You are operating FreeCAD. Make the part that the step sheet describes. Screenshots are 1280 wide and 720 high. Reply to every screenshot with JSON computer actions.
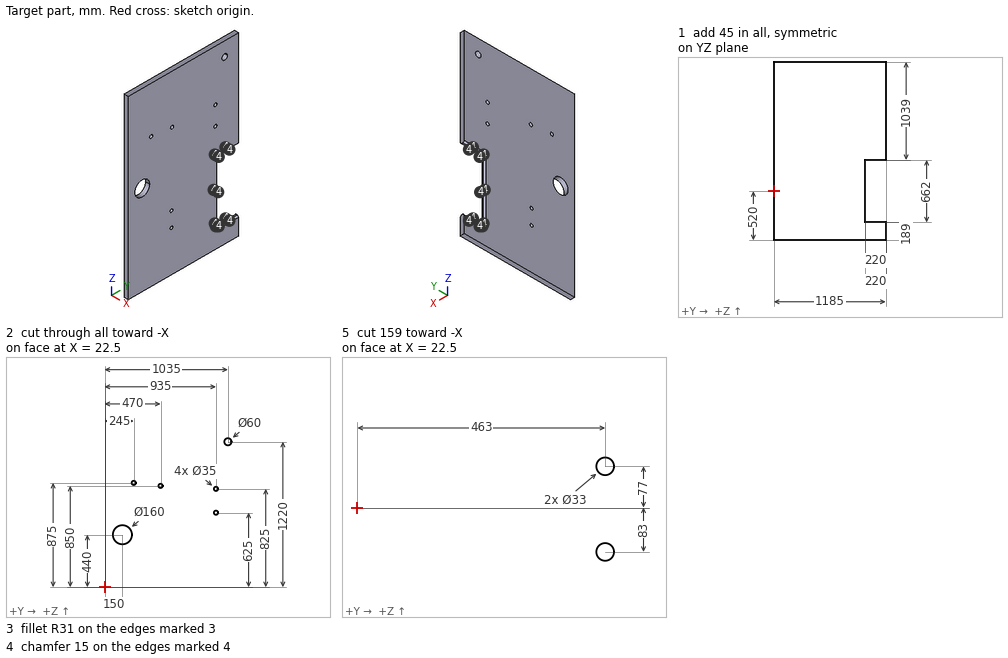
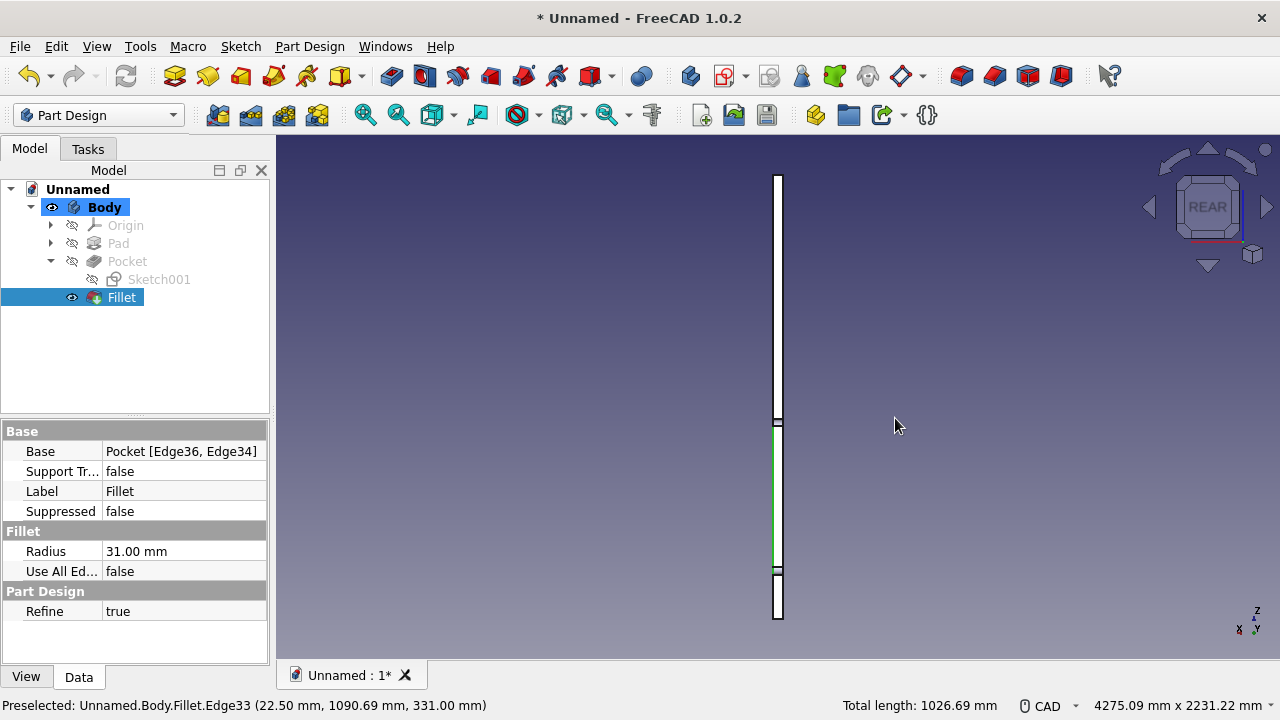
{"action": "left_click", "coordinate": [783, 496], "text": "ctrl"}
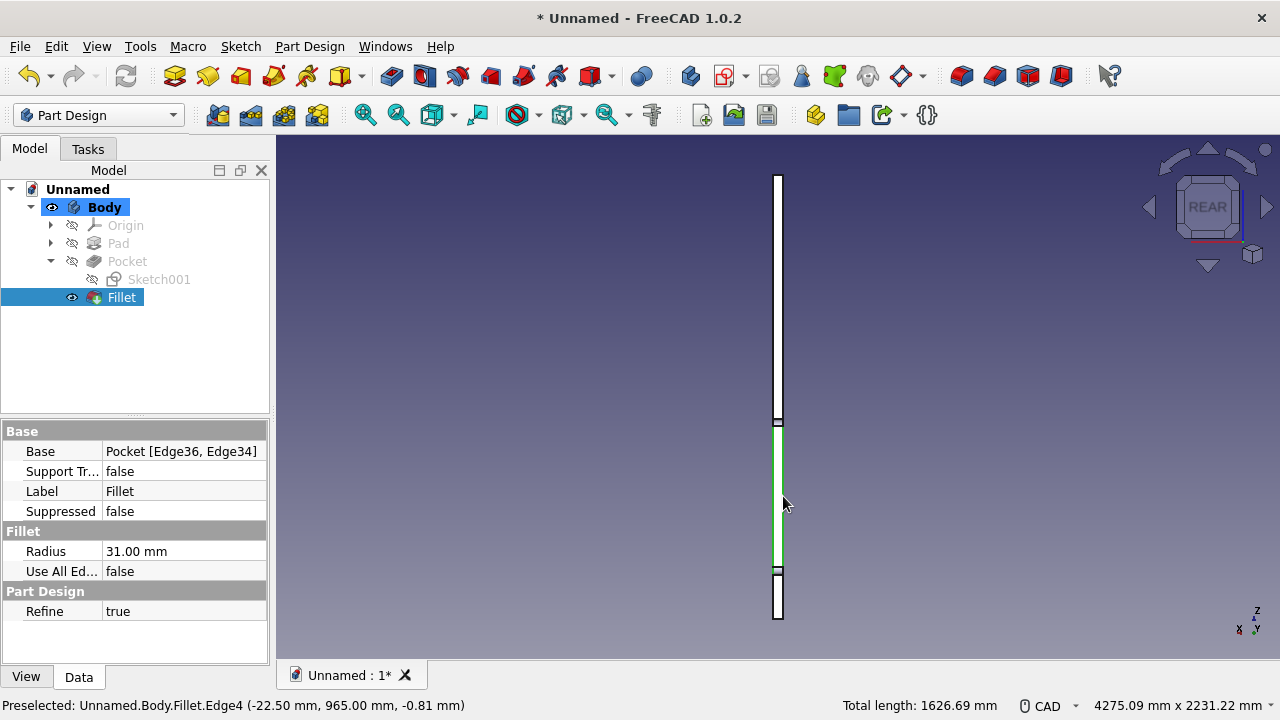
{"action": "left_click", "coordinate": [783, 425], "text": "ctrl"}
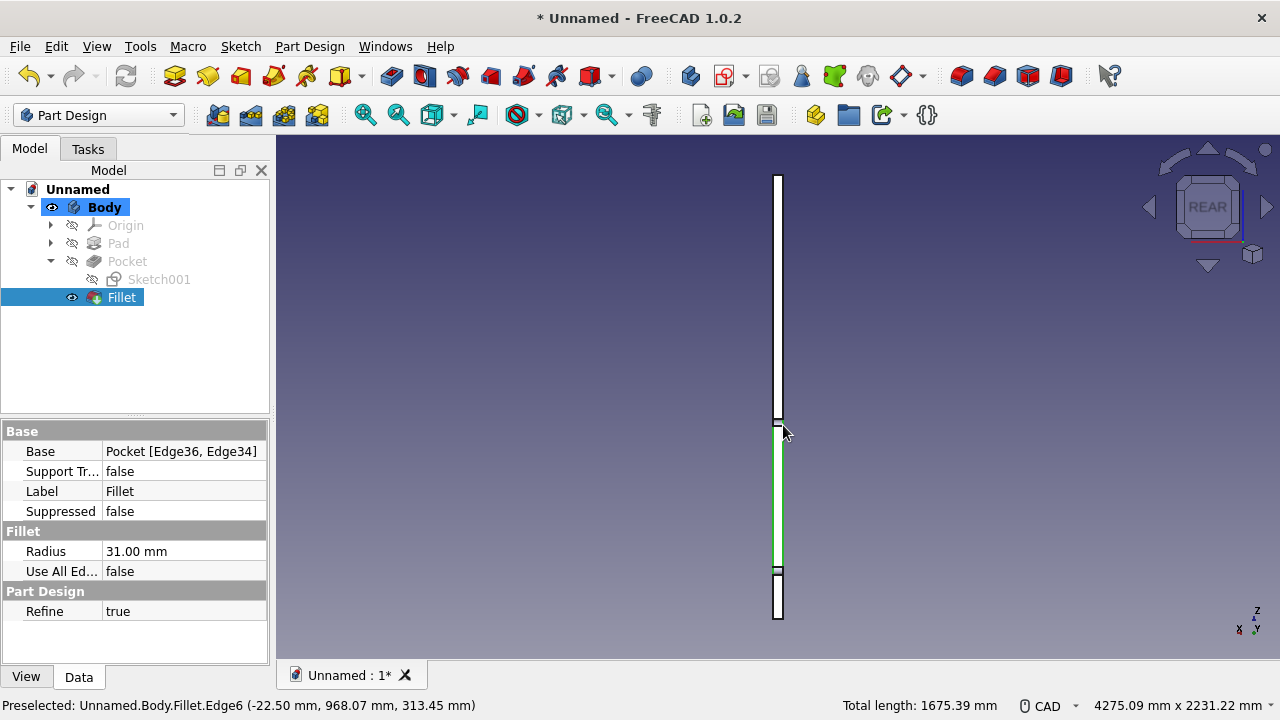
{"action": "left_click", "coordinate": [773, 425], "text": "ctrl"}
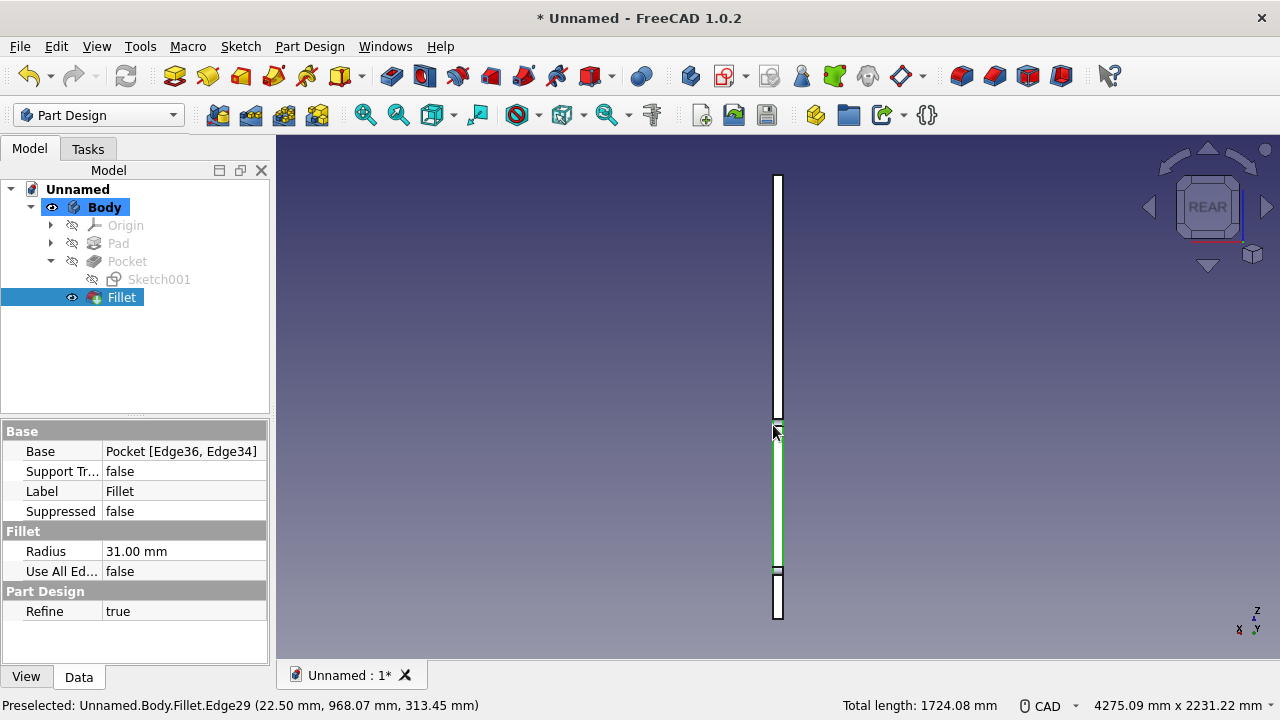
{"action": "key", "text": "6"}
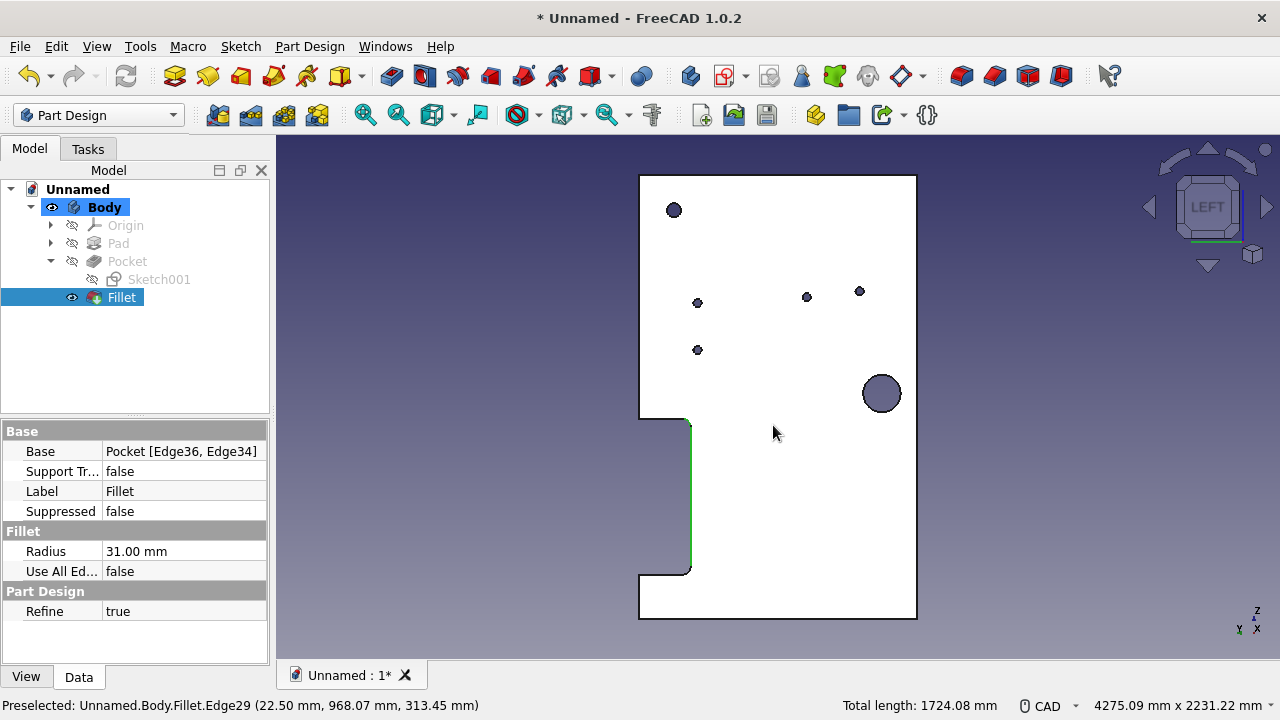
{"action": "left_click", "coordinate": [661, 574], "text": "ctrl"}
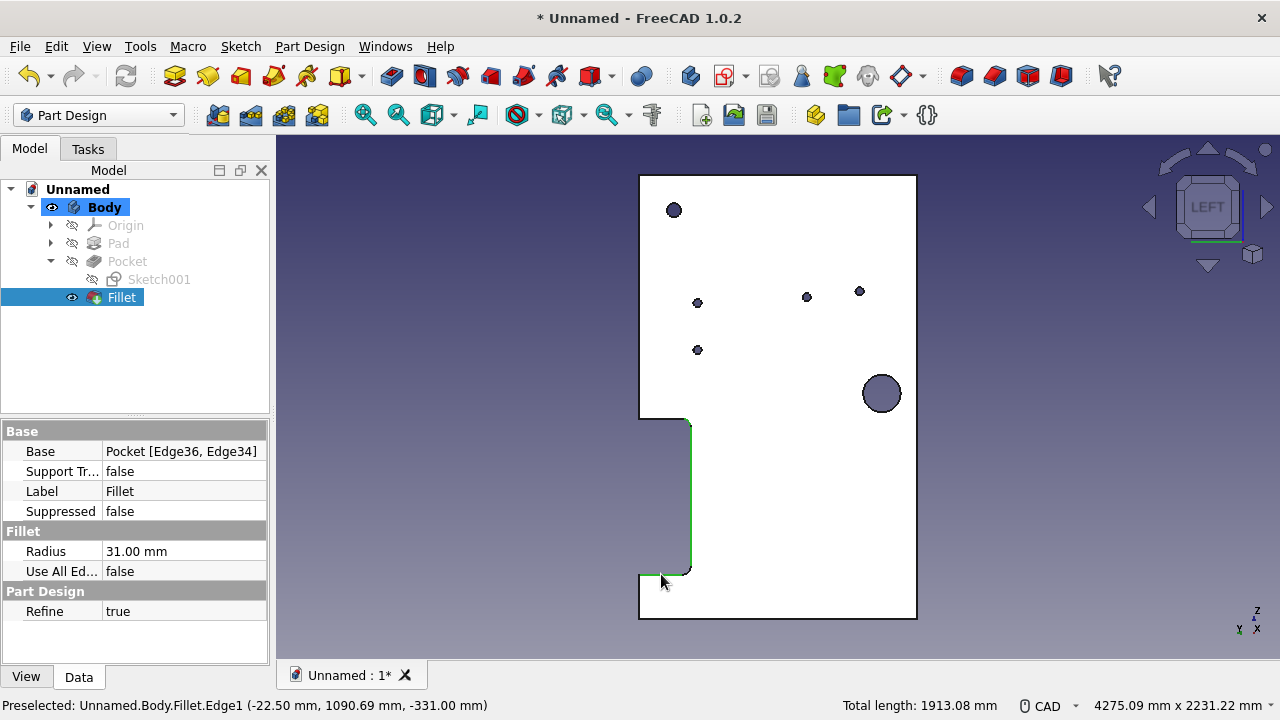
{"action": "left_click", "coordinate": [661, 418], "text": "ctrl"}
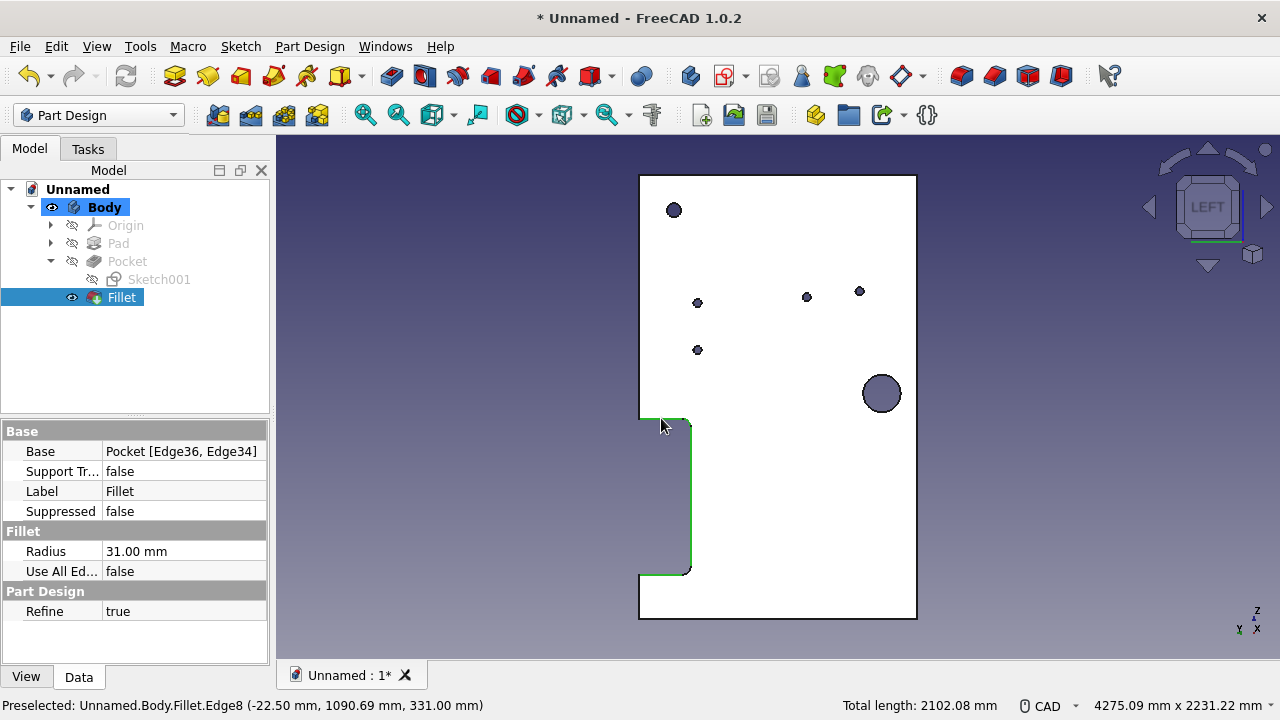
{"action": "scroll", "coordinate": [688, 571], "scroll_direction": "up", "scroll_amount": 7}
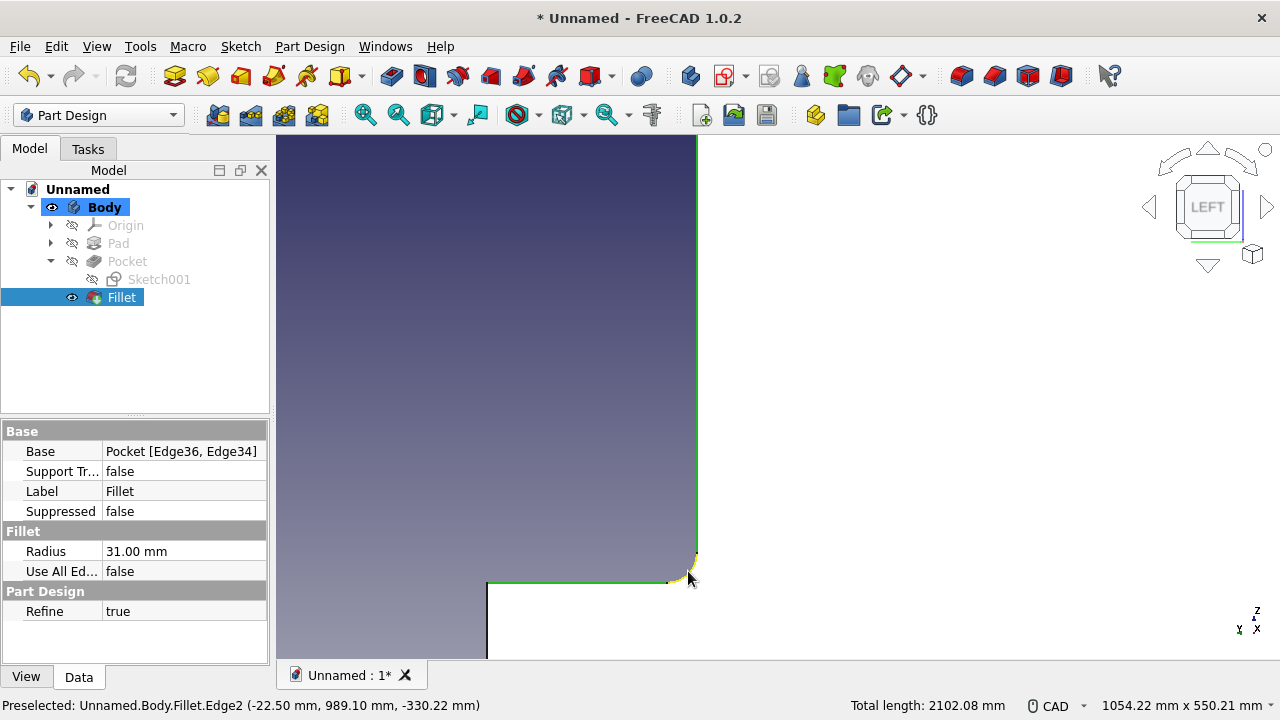
{"action": "left_click", "coordinate": [688, 573], "text": "ctrl"}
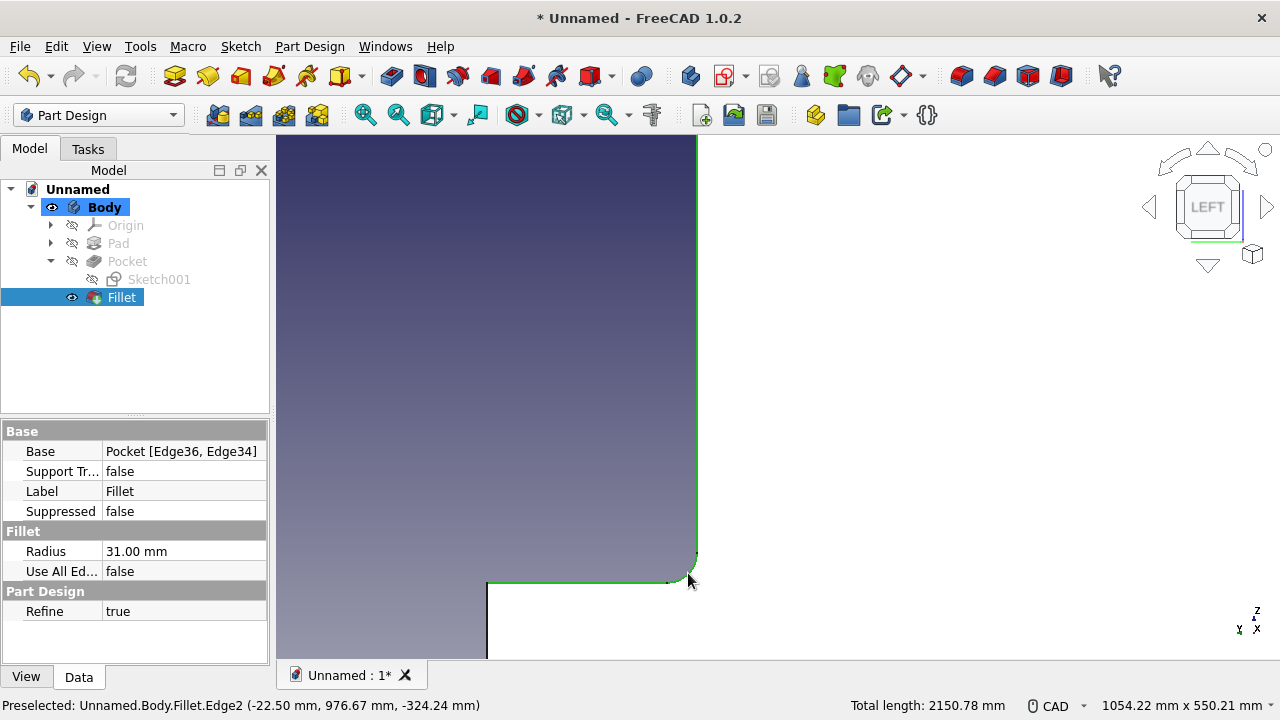
{"action": "left_click", "coordinate": [995, 76]}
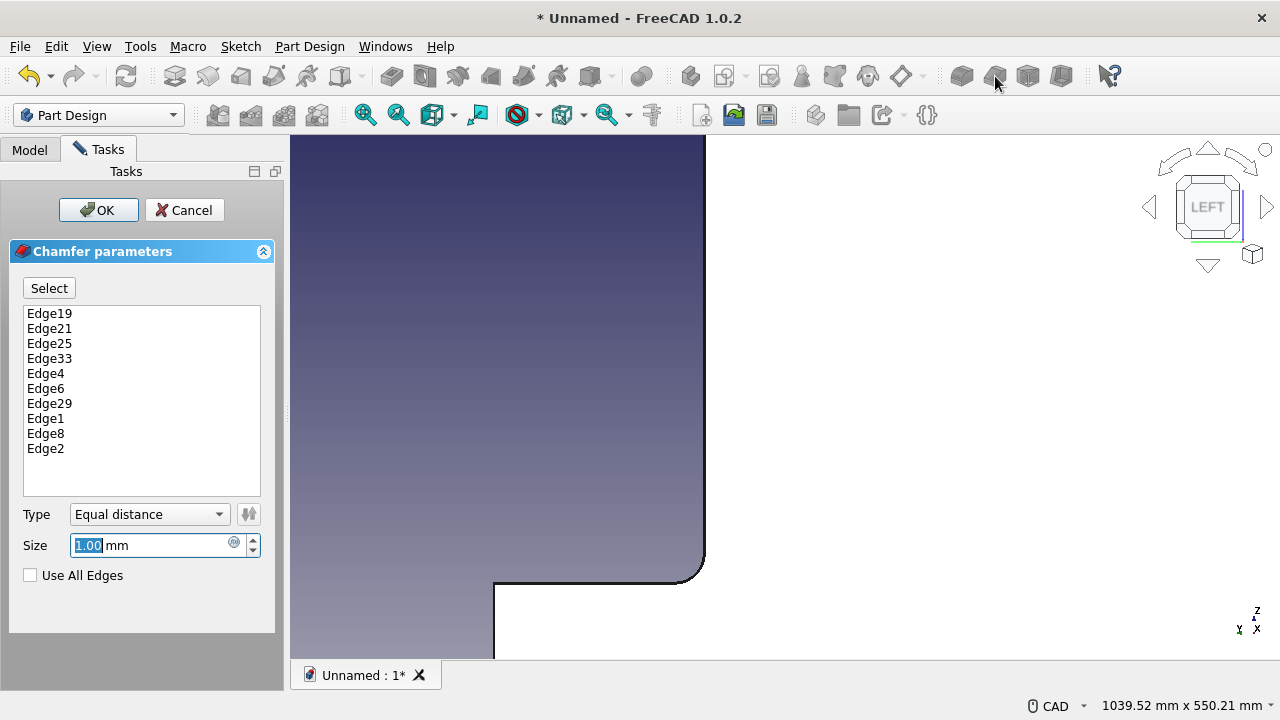
{"action": "type", "text": "15"}
{"action": "key", "text": "Tab"}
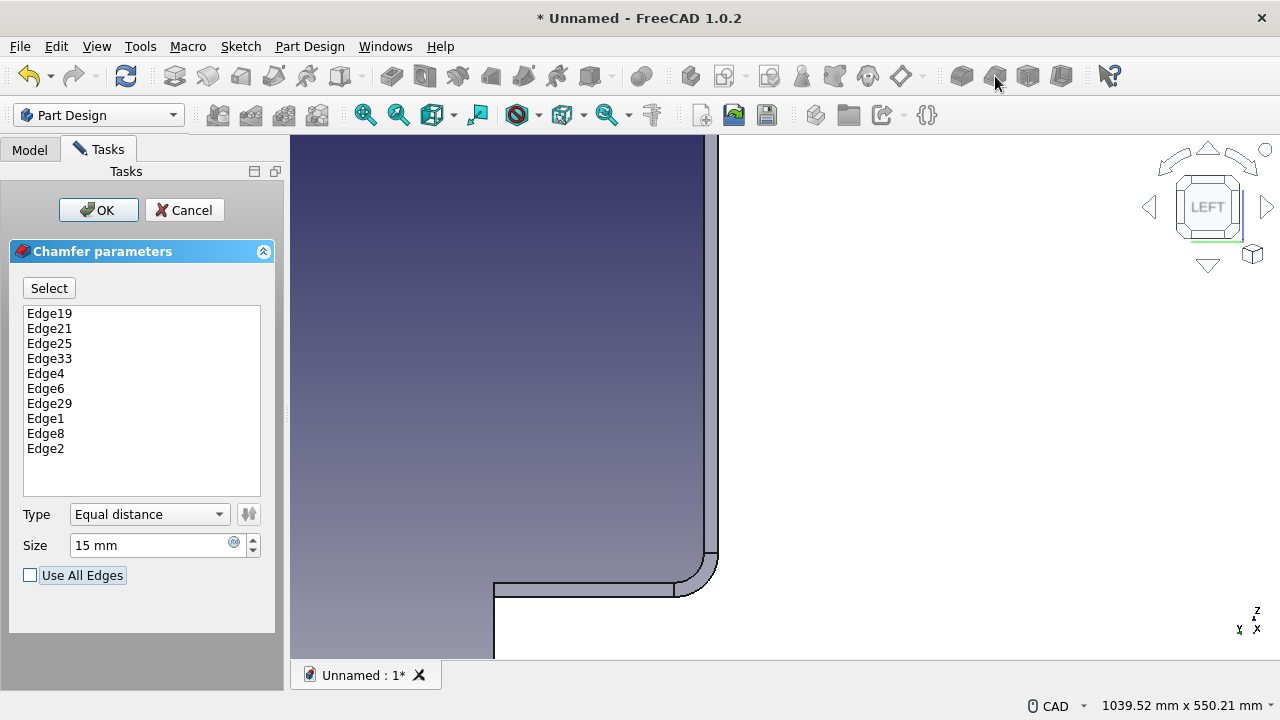
{"action": "left_click", "coordinate": [99, 210]}